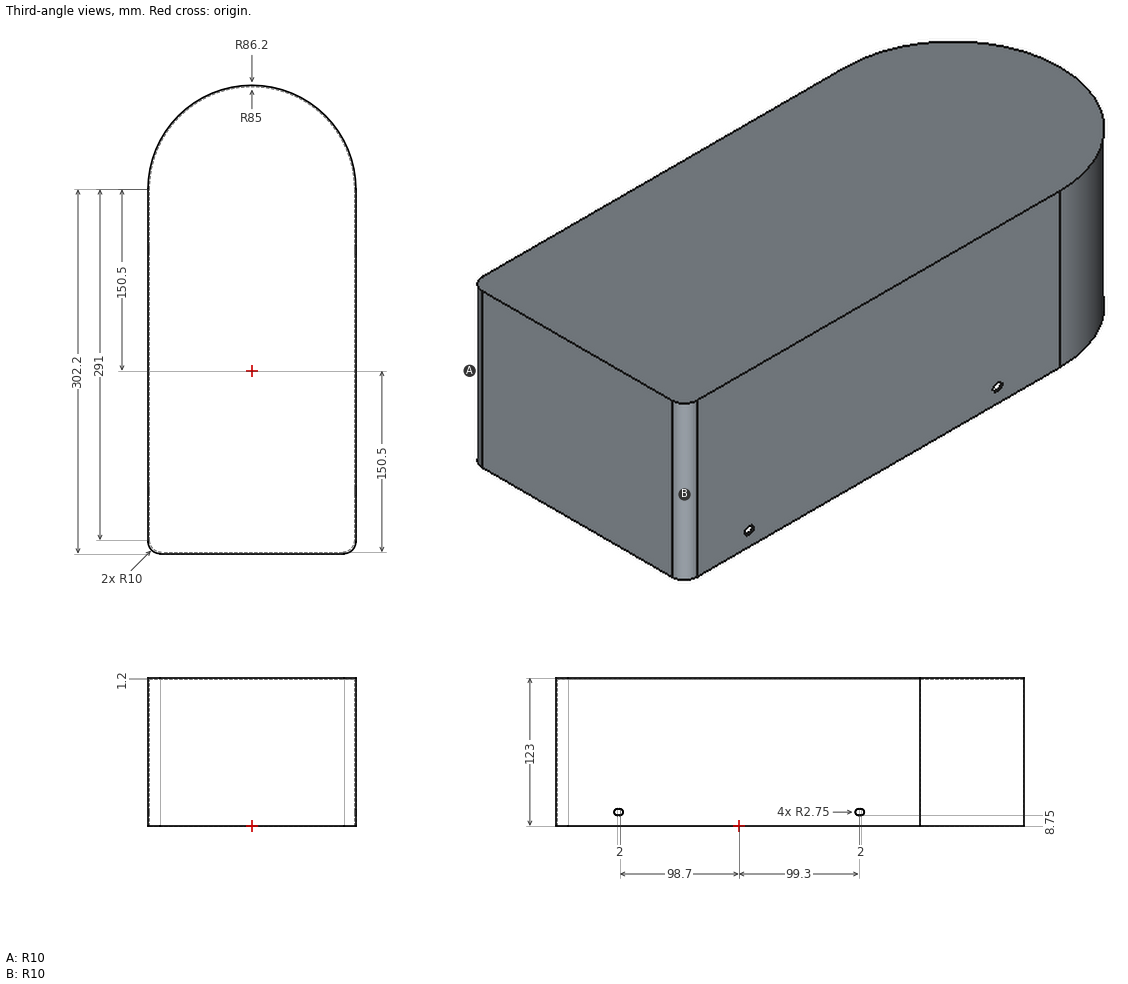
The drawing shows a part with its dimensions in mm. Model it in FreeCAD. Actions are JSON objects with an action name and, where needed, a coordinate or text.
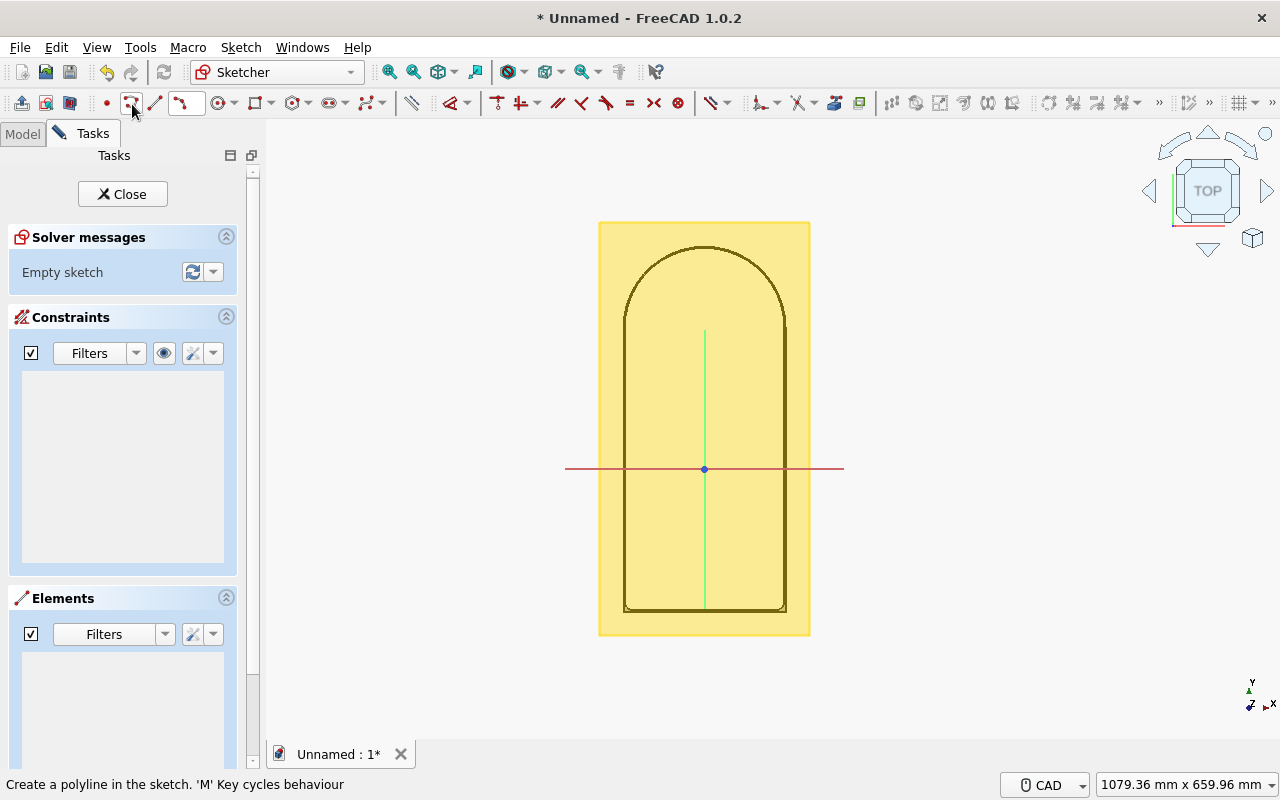
{"action": "left_click", "coordinate": [624, 328]}
{"action": "left_click", "coordinate": [624, 612]}
{"action": "left_click", "coordinate": [786, 612]}
{"action": "left_click", "coordinate": [786, 328]}
{"action": "right_click", "coordinate": [786, 328]}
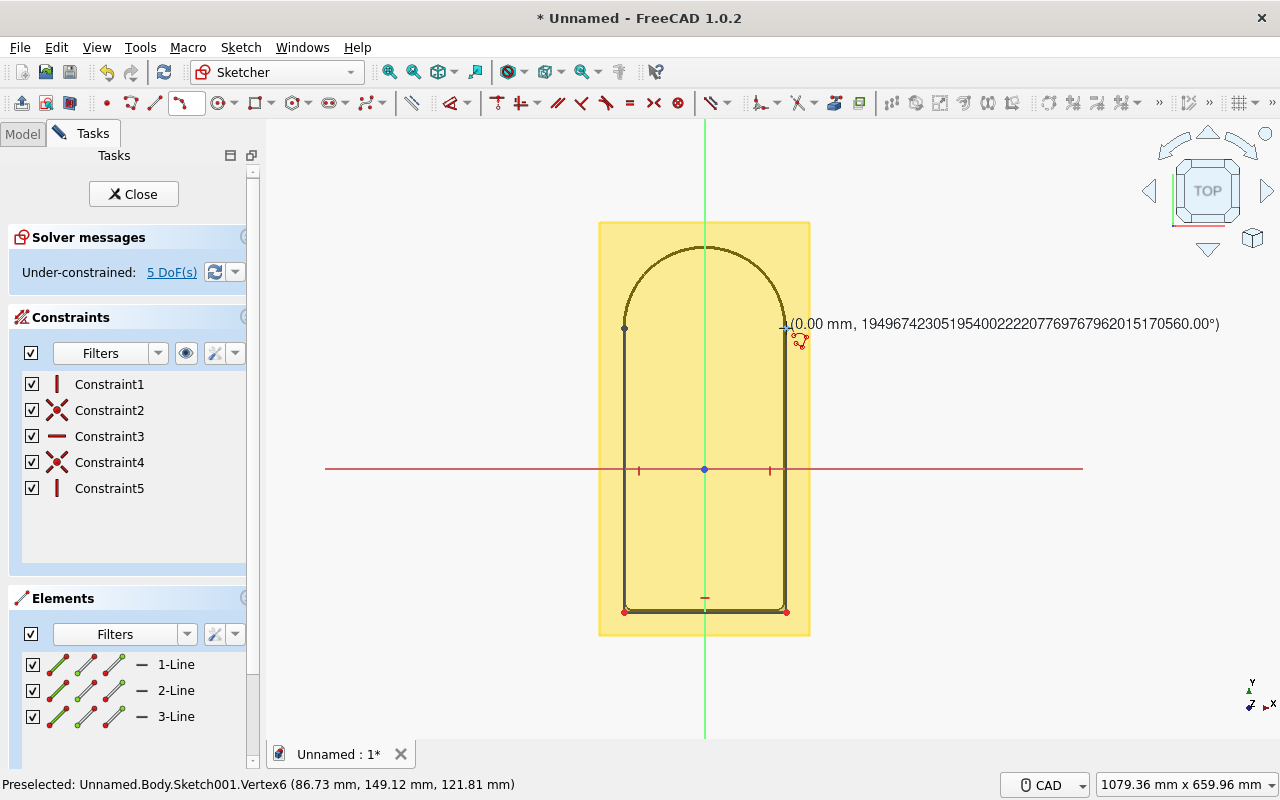
{"action": "left_click", "coordinate": [180, 104]}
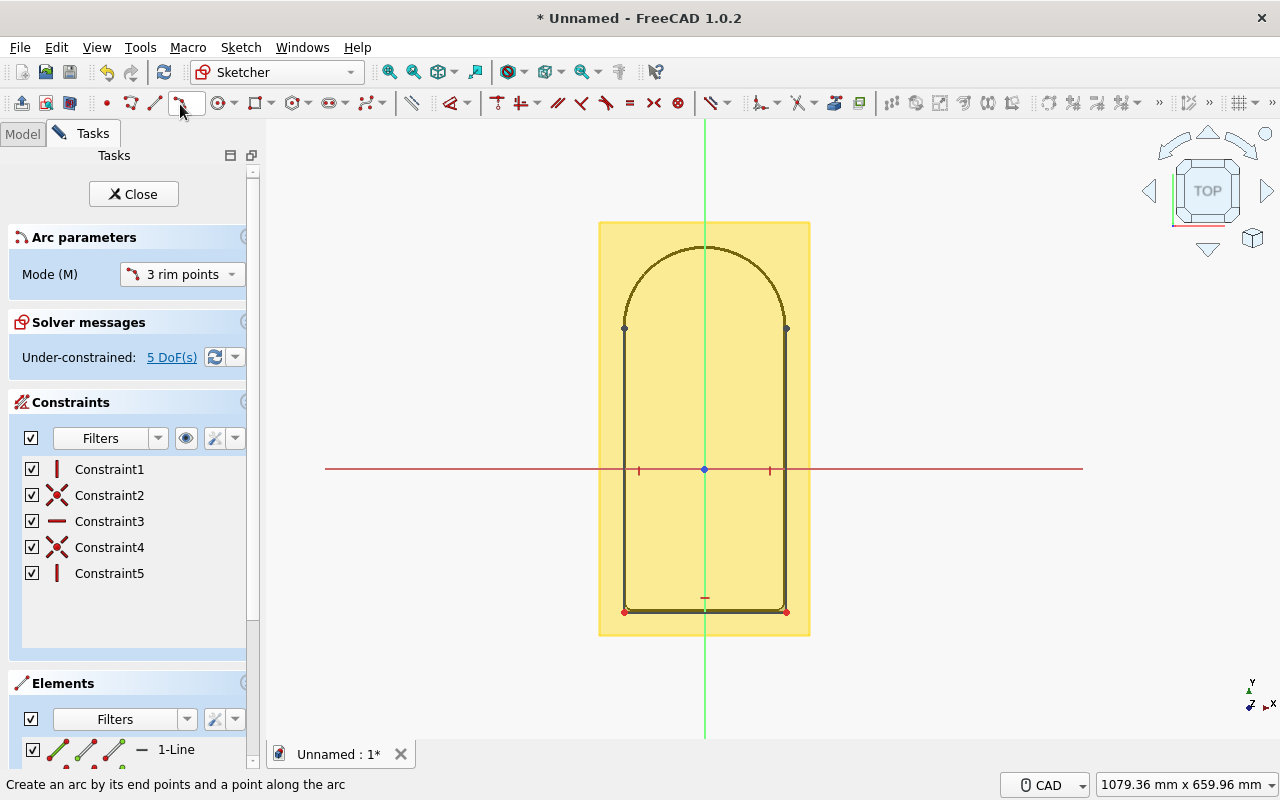
{"action": "left_click", "coordinate": [786, 329]}
{"action": "left_click", "coordinate": [624, 329]}
{"action": "left_click", "coordinate": [730, 251]}
{"action": "key", "text": "Escape"}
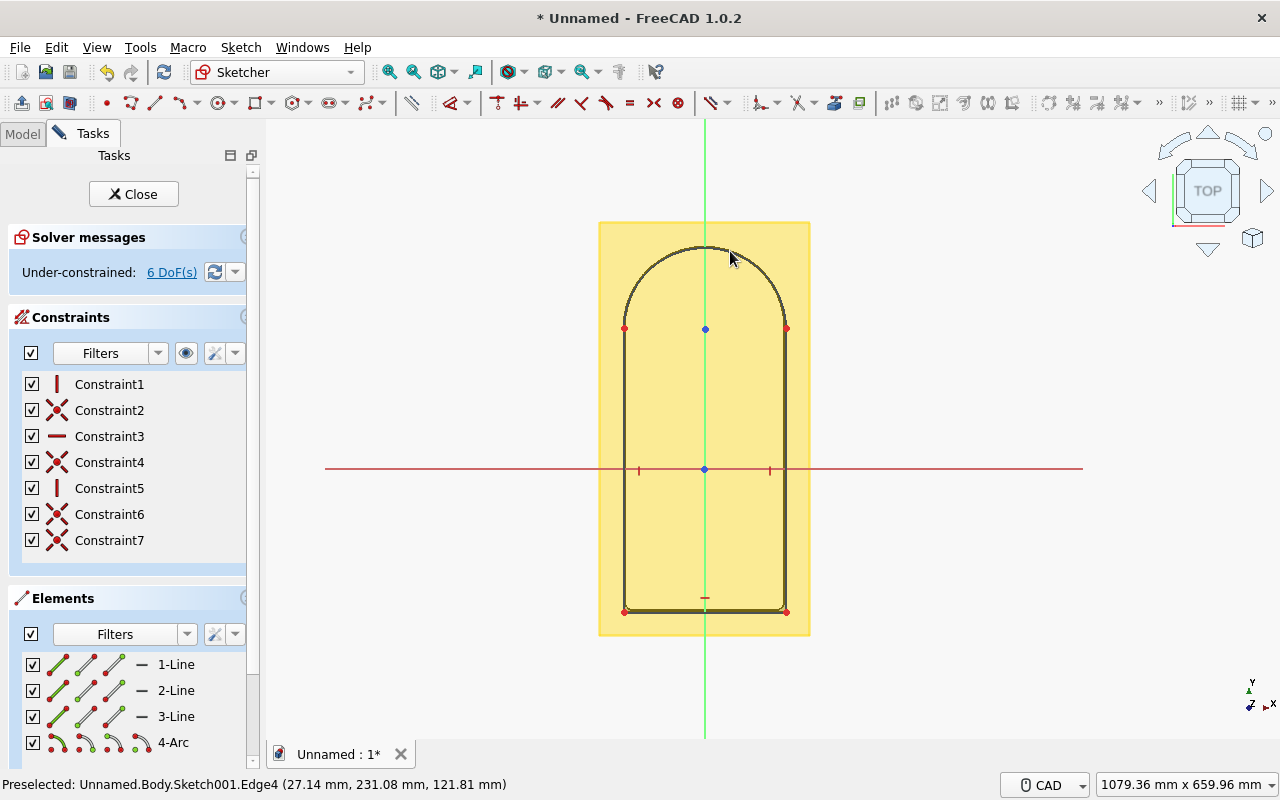
{"action": "left_click", "coordinate": [705, 329]}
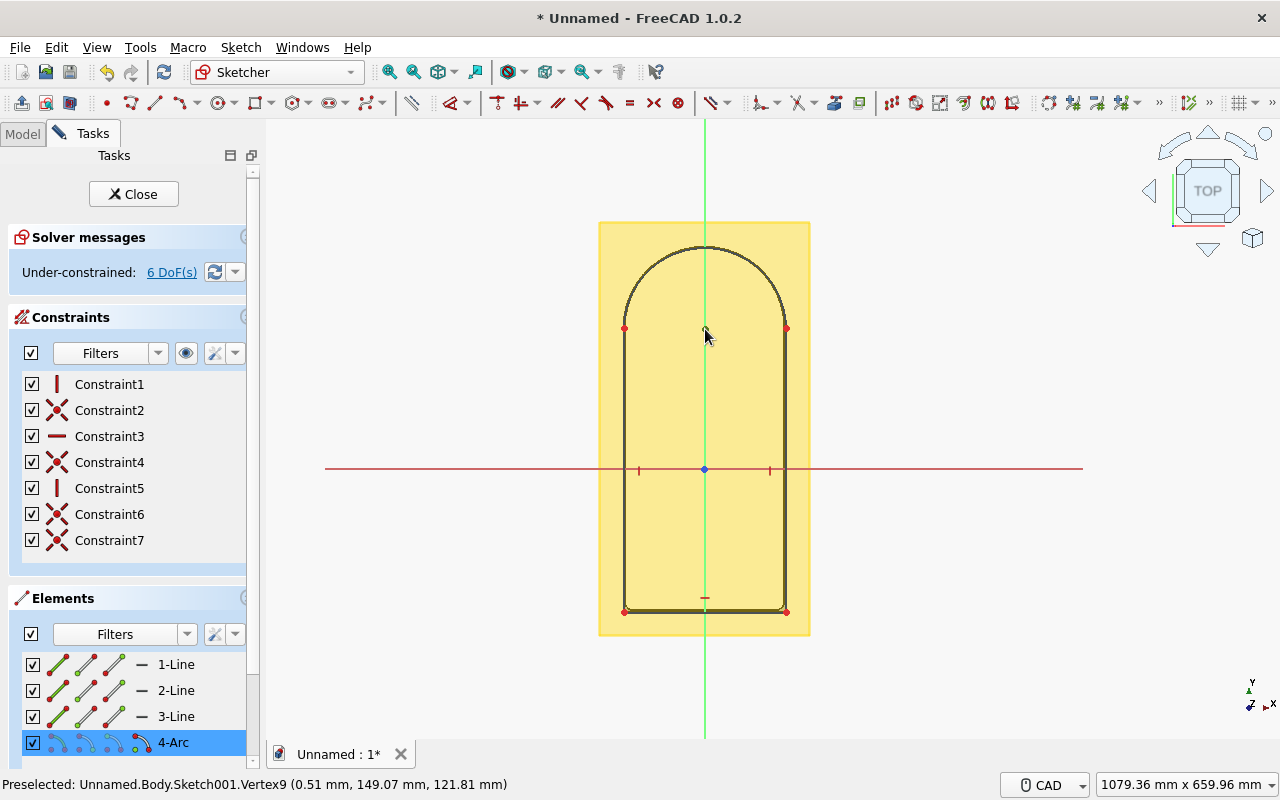
{"action": "left_click", "coordinate": [705, 671]}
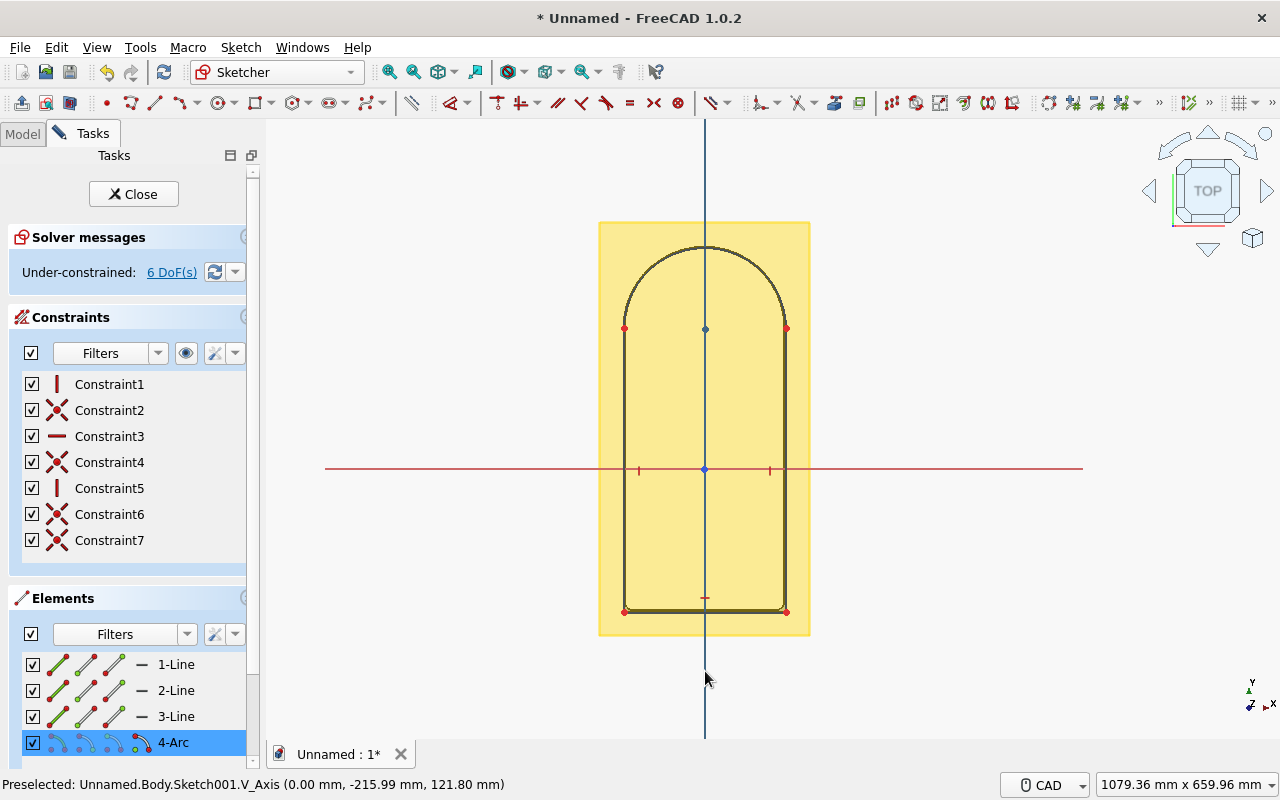
{"action": "left_click", "coordinate": [498, 104]}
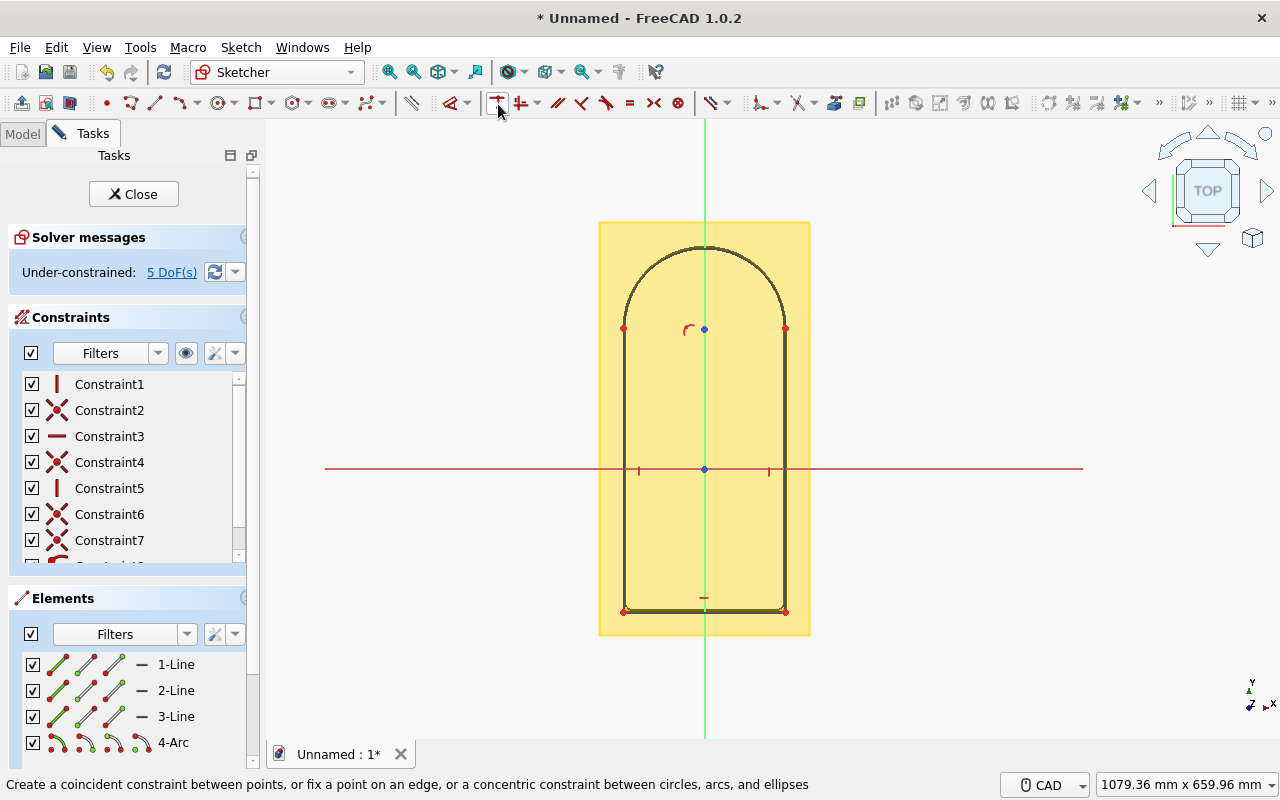
{"action": "key", "text": "d"}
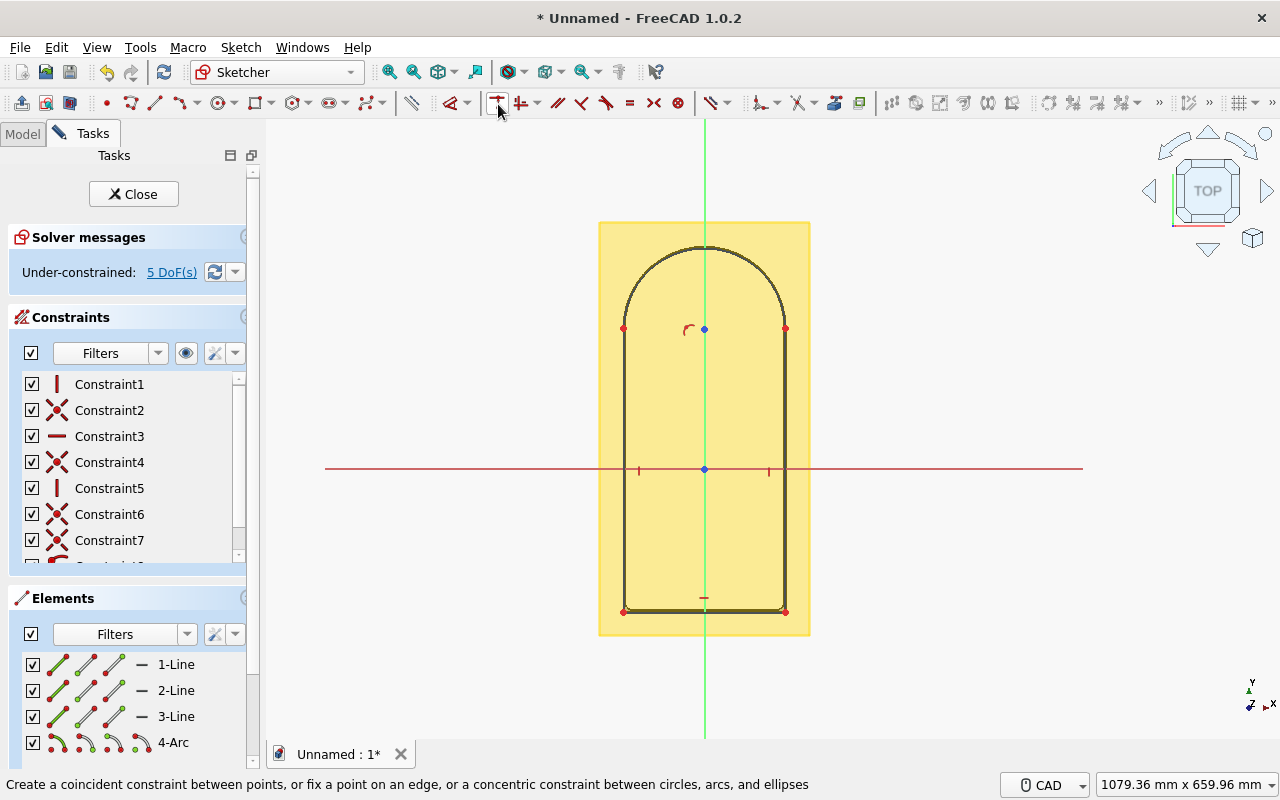
{"action": "left_click", "coordinate": [752, 264]}
{"action": "left_click", "coordinate": [771, 238]}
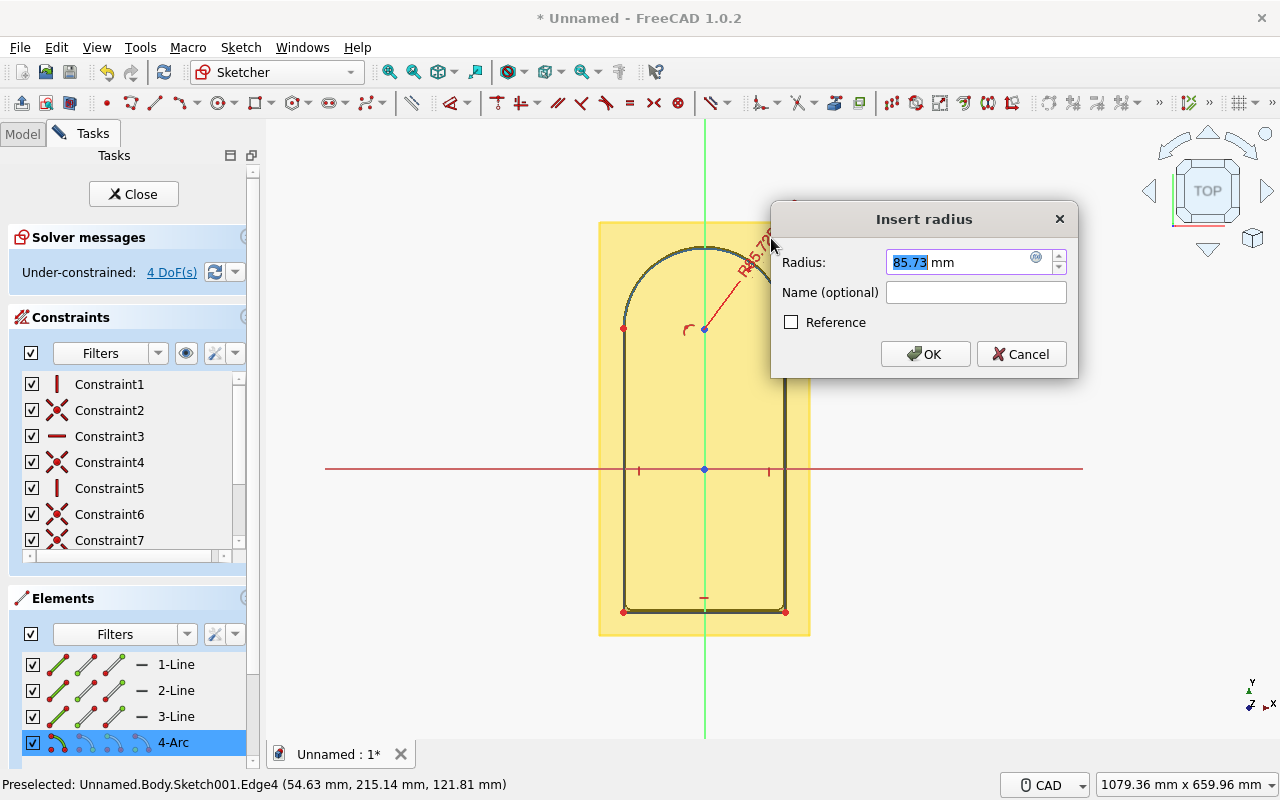
{"action": "type", "text": "86.2"}
{"action": "key", "text": "Return"}